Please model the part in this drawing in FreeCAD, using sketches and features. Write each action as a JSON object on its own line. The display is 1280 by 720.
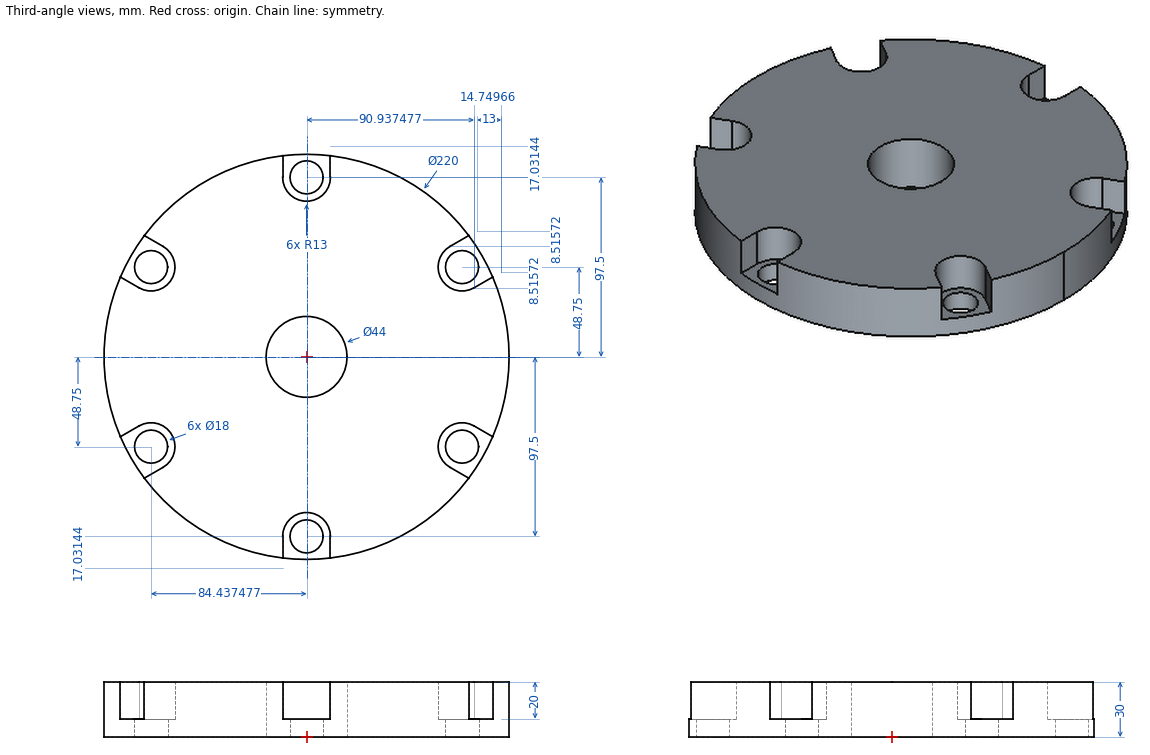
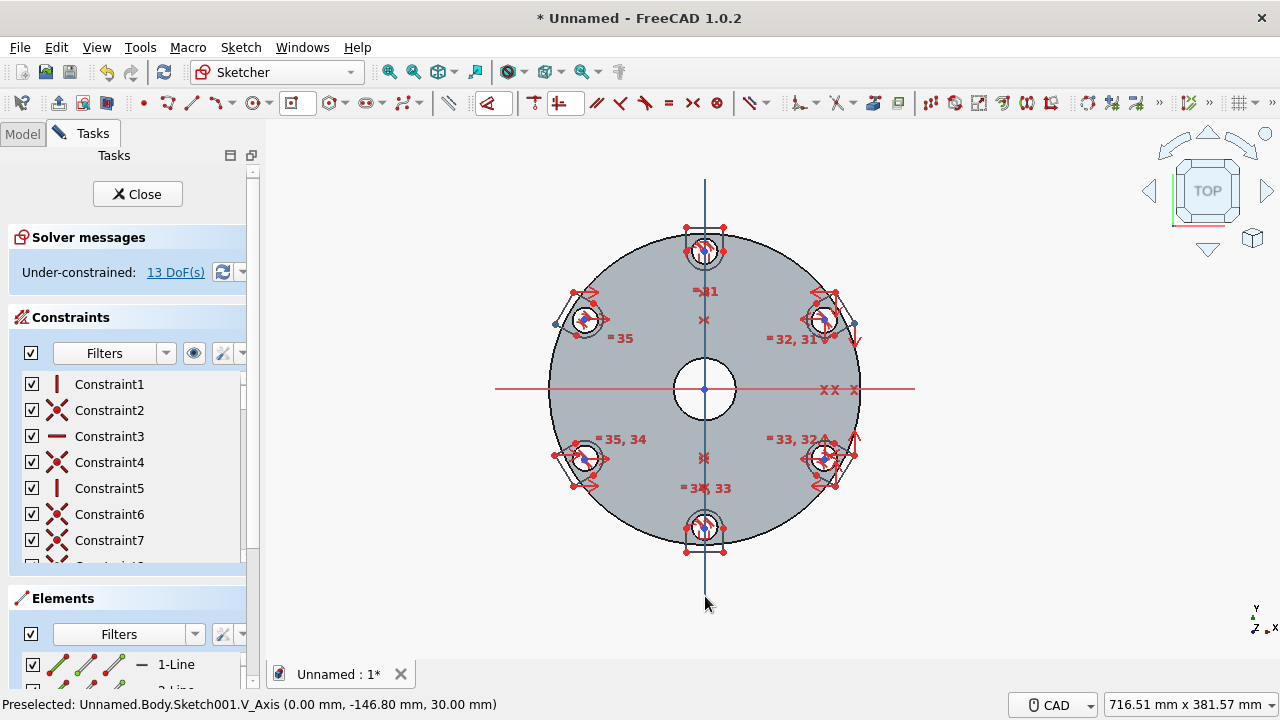
{"action": "left_click", "coordinate": [694, 104]}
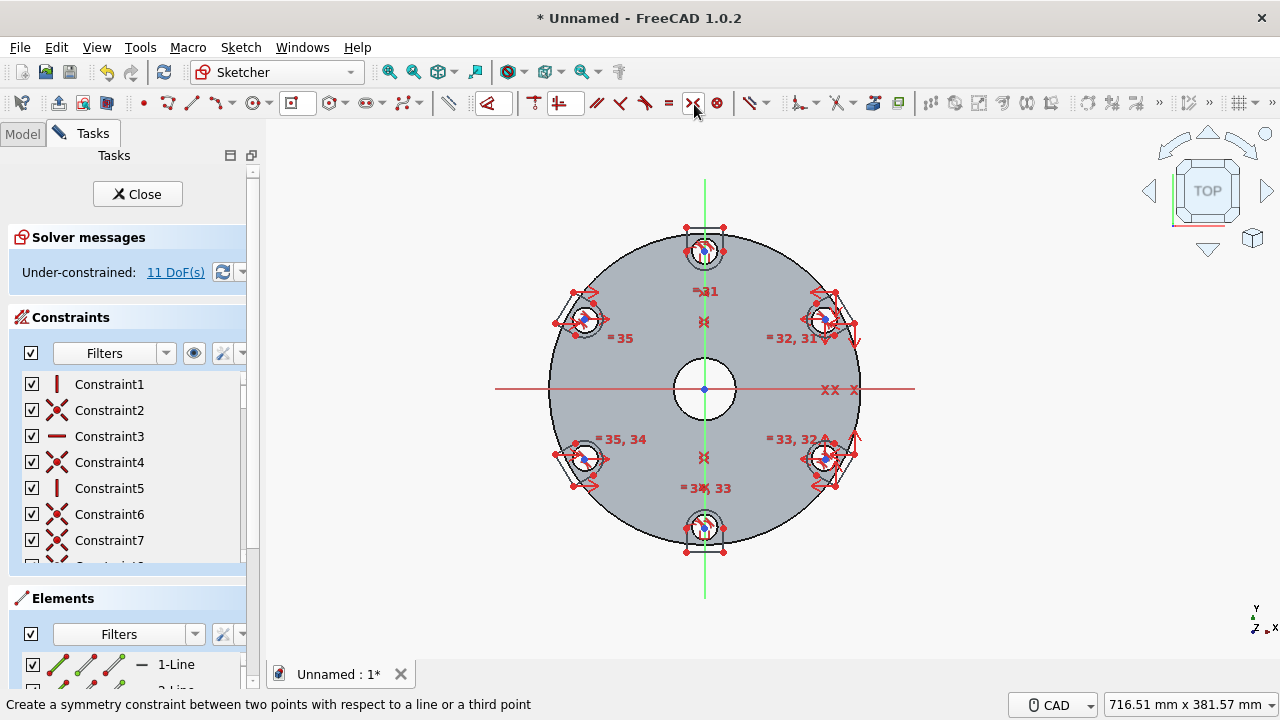
{"action": "scroll", "coordinate": [694, 267], "scroll_direction": "up", "scroll_amount": 4}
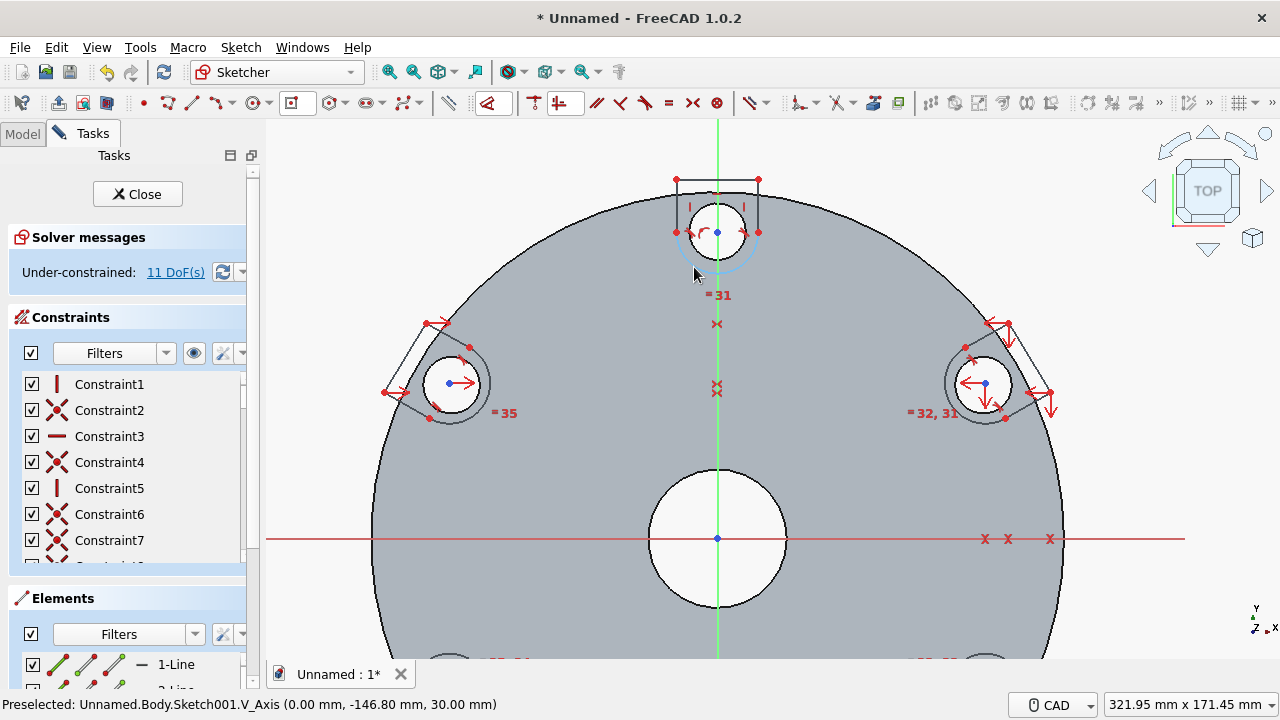
{"action": "left_click", "coordinate": [694, 266]}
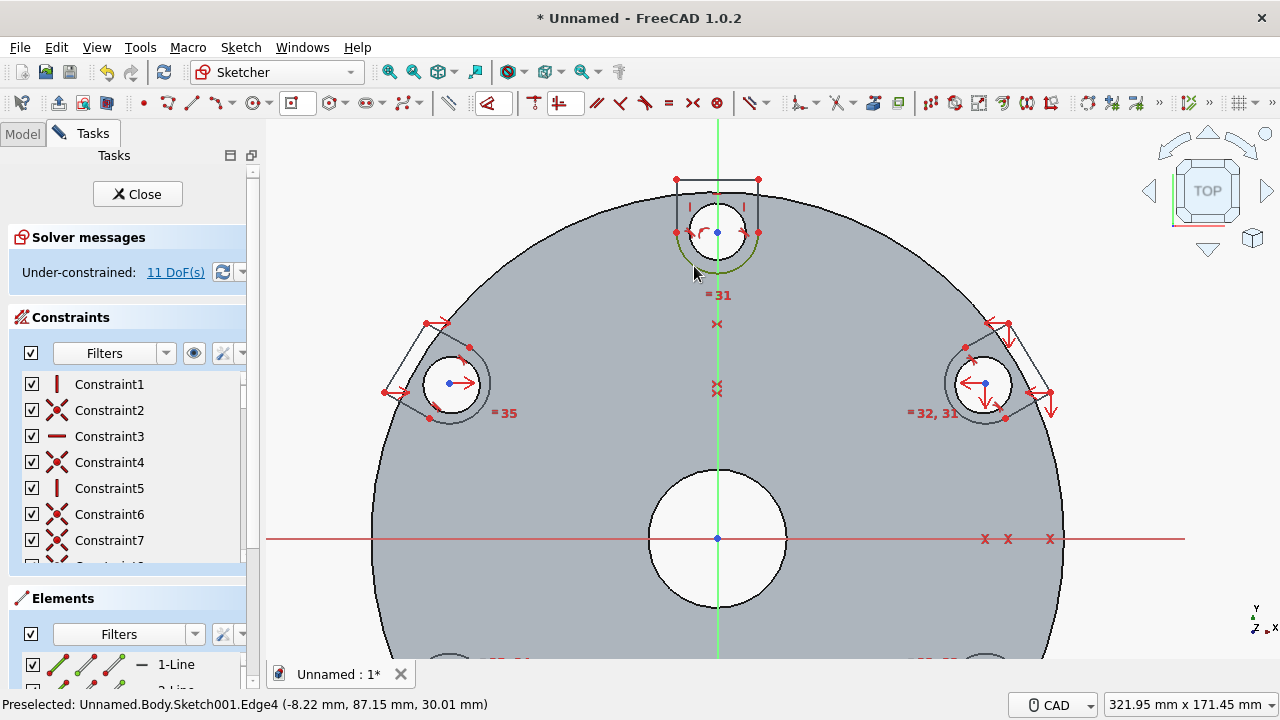
{"action": "left_click", "coordinate": [506, 104]}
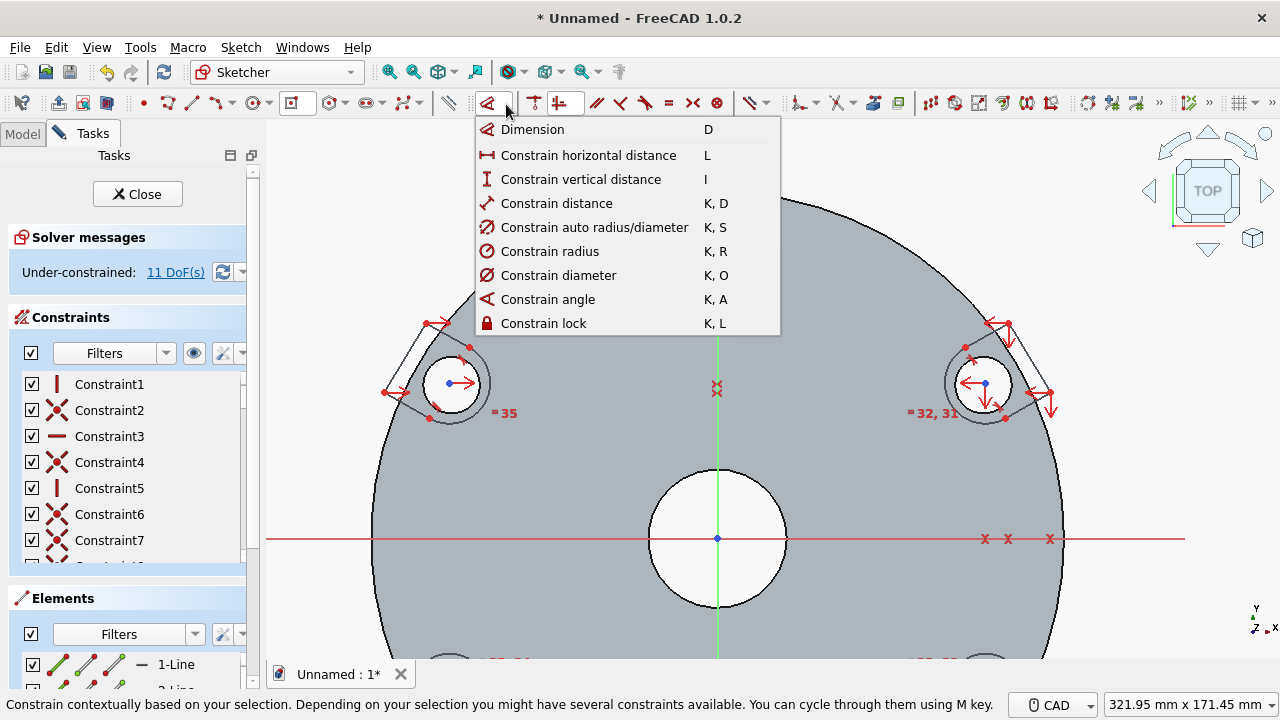
{"action": "left_click", "coordinate": [628, 251]}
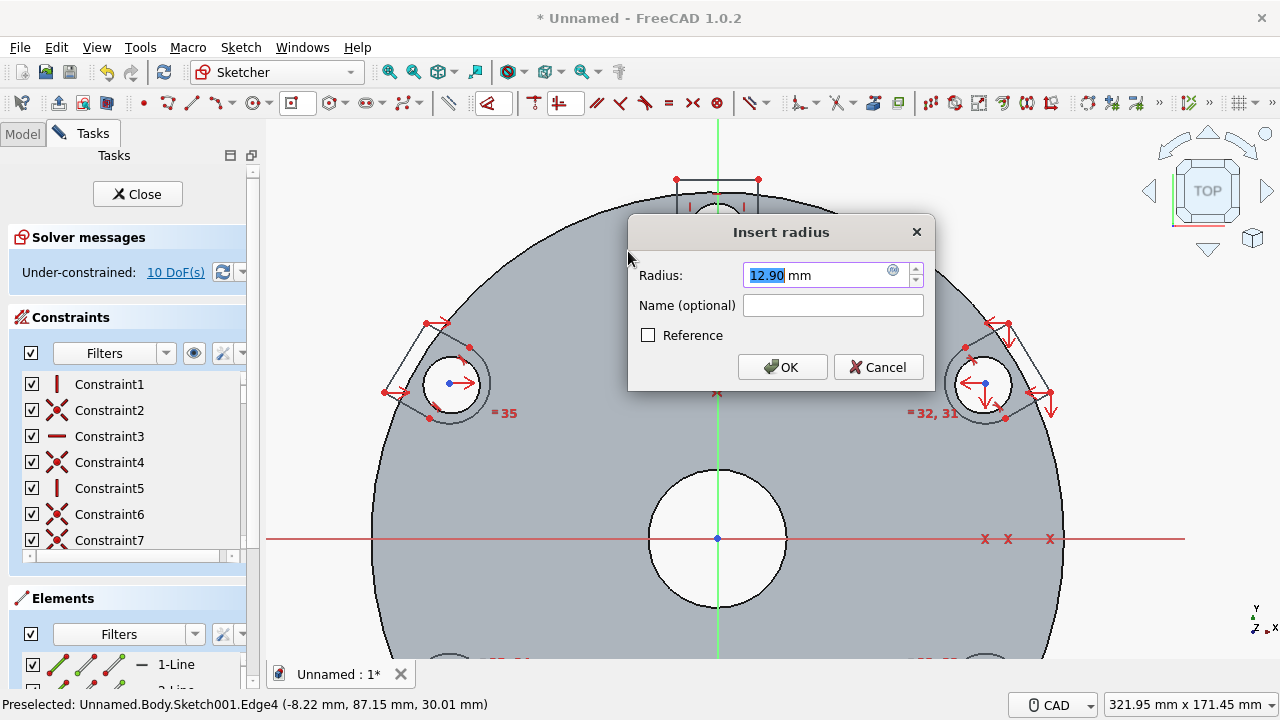
{"action": "type", "text": "13"}
{"action": "key", "text": "Return"}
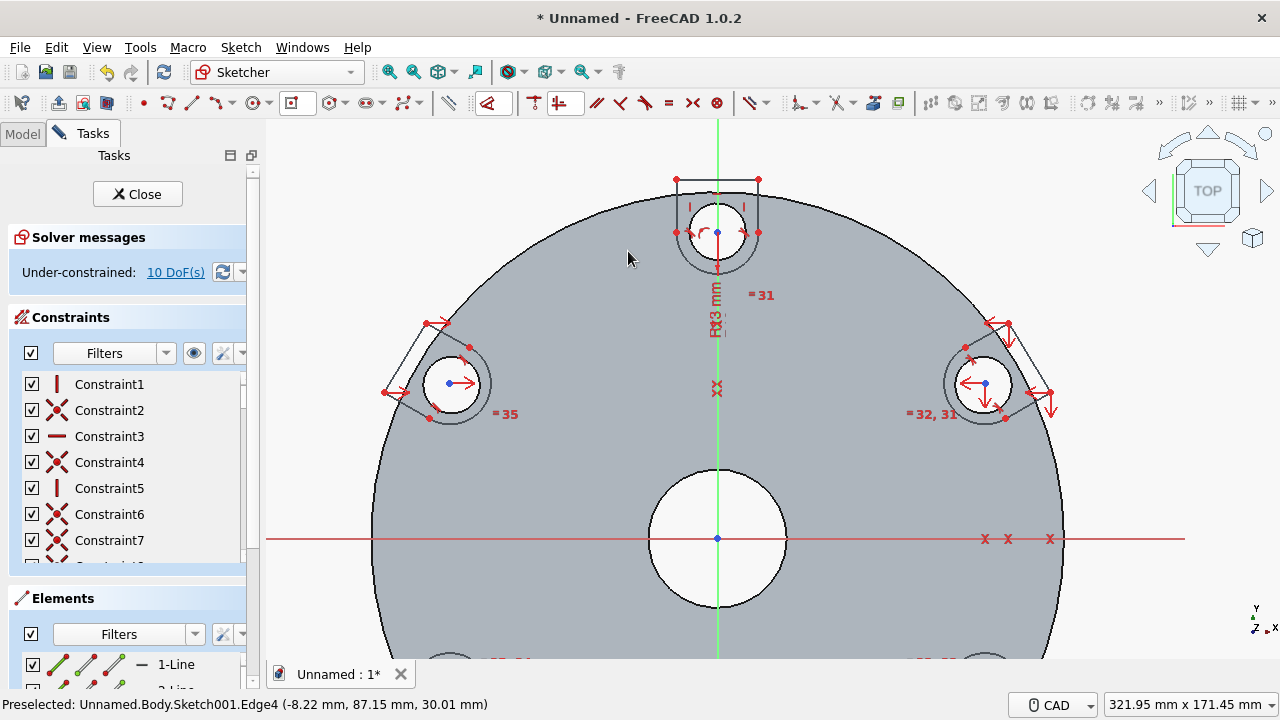
{"action": "left_click", "coordinate": [1038, 372]}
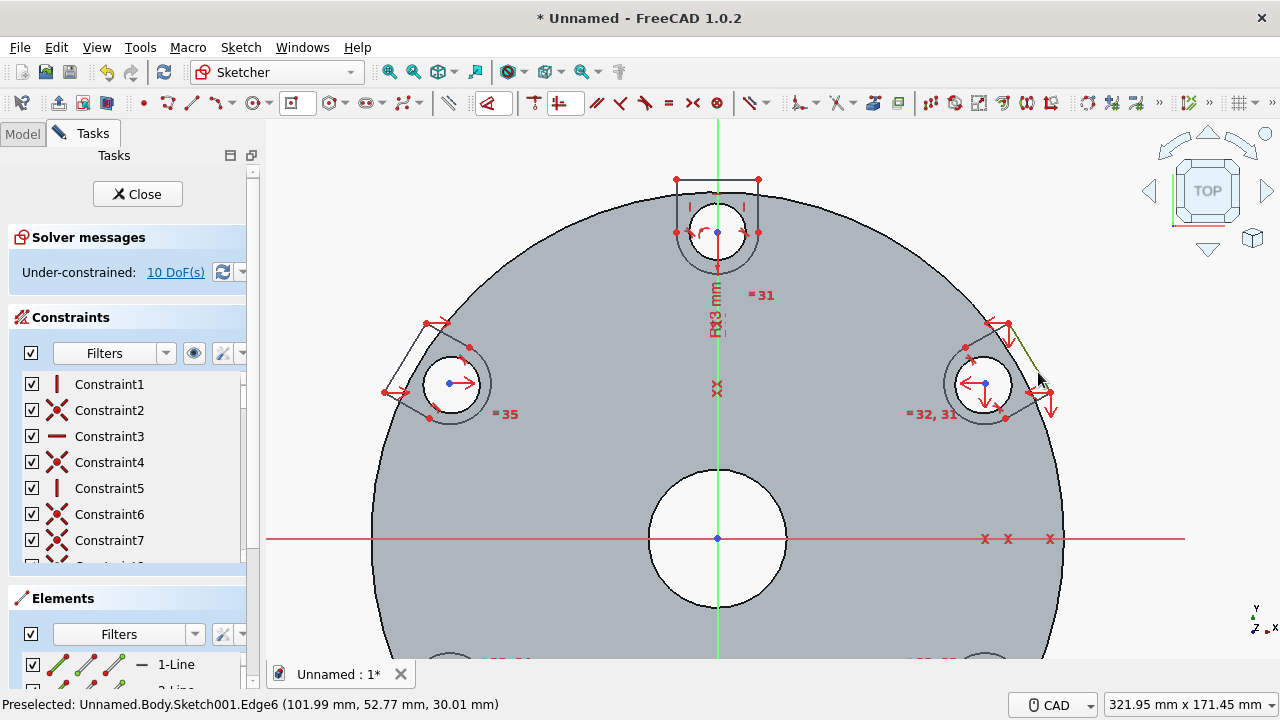
{"action": "key", "text": "l"}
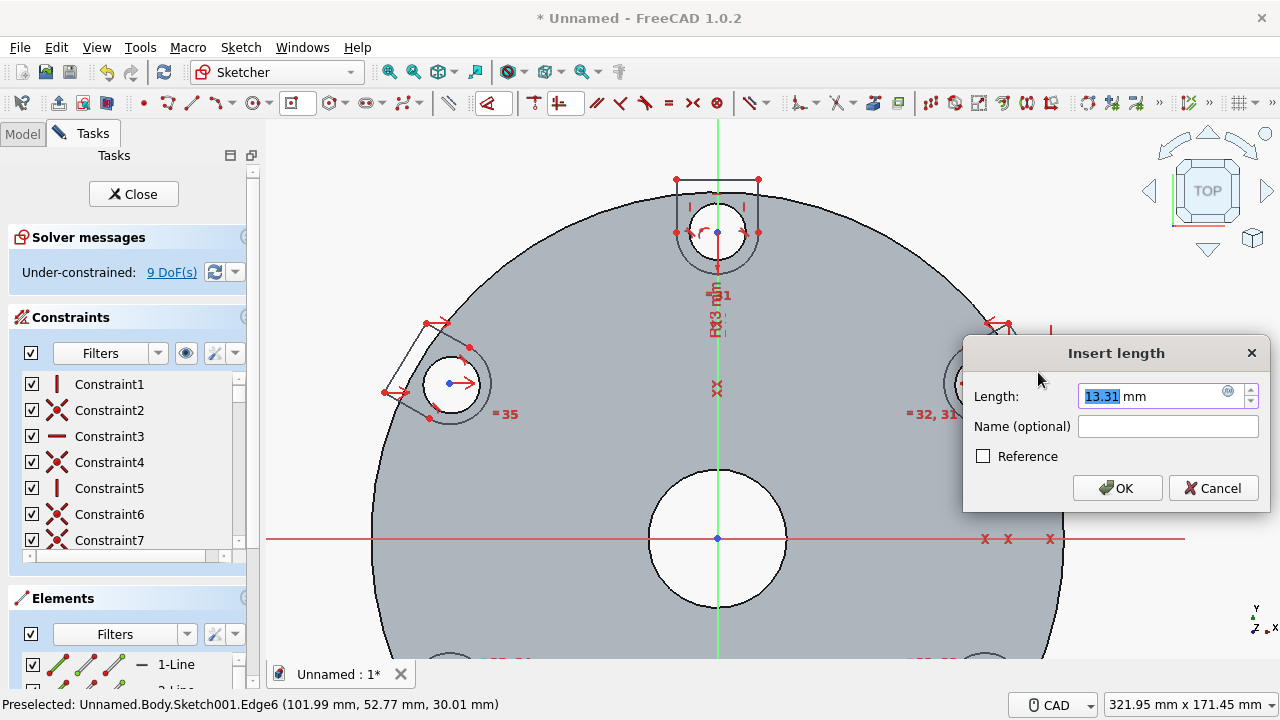
{"action": "type", "text": "13"}
{"action": "key", "text": "Return"}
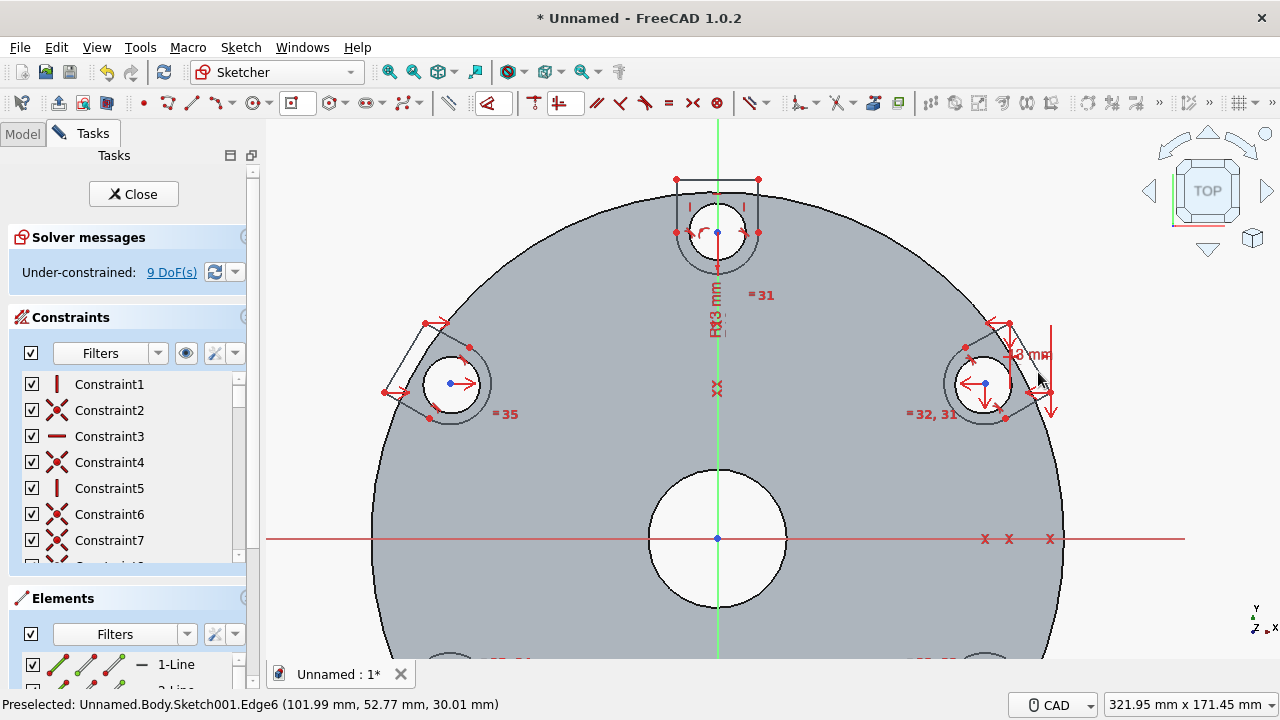
{"action": "left_click", "coordinate": [758, 233]}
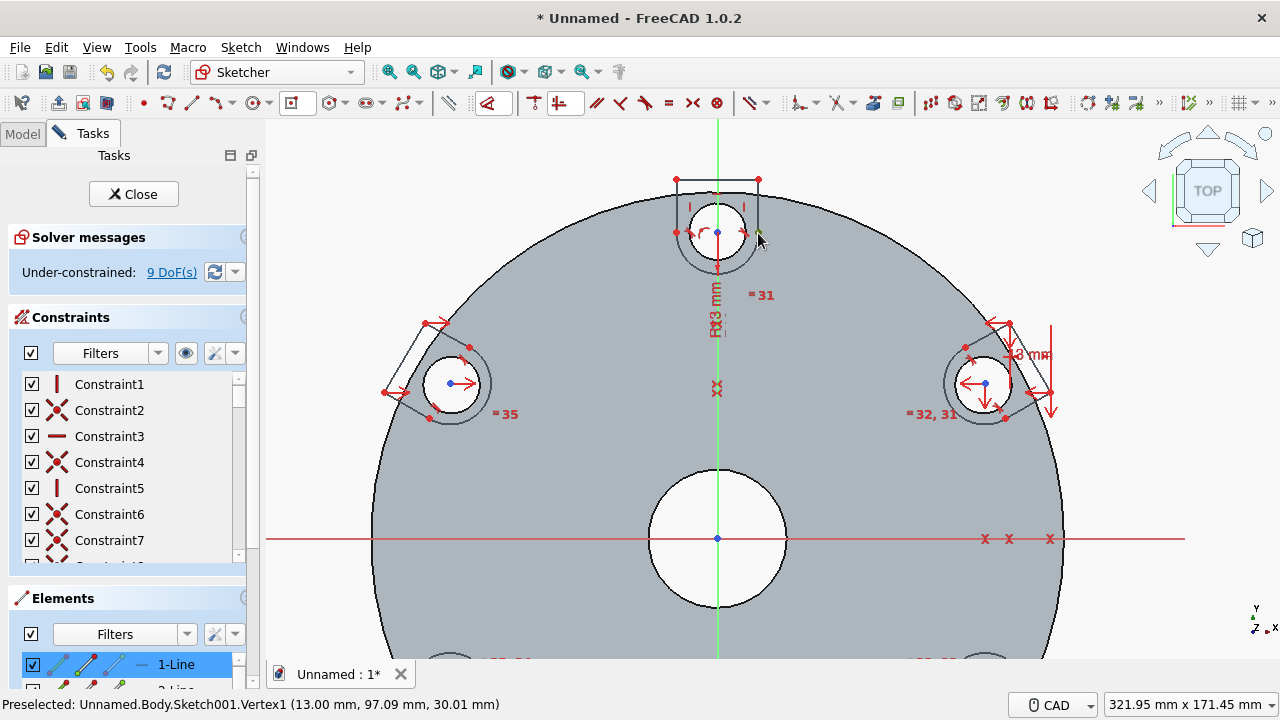
{"action": "left_click", "coordinate": [506, 104]}